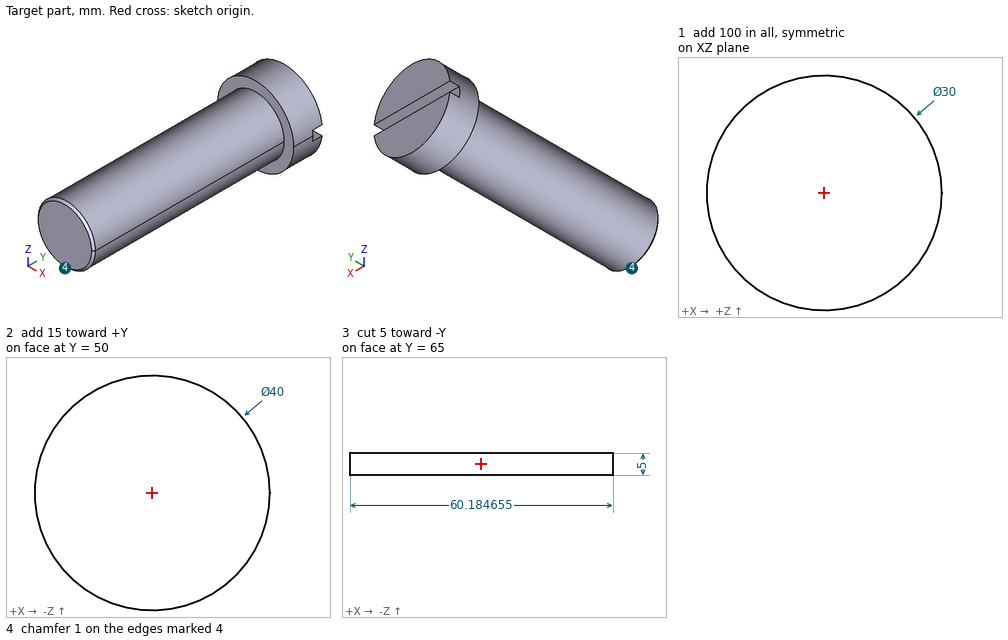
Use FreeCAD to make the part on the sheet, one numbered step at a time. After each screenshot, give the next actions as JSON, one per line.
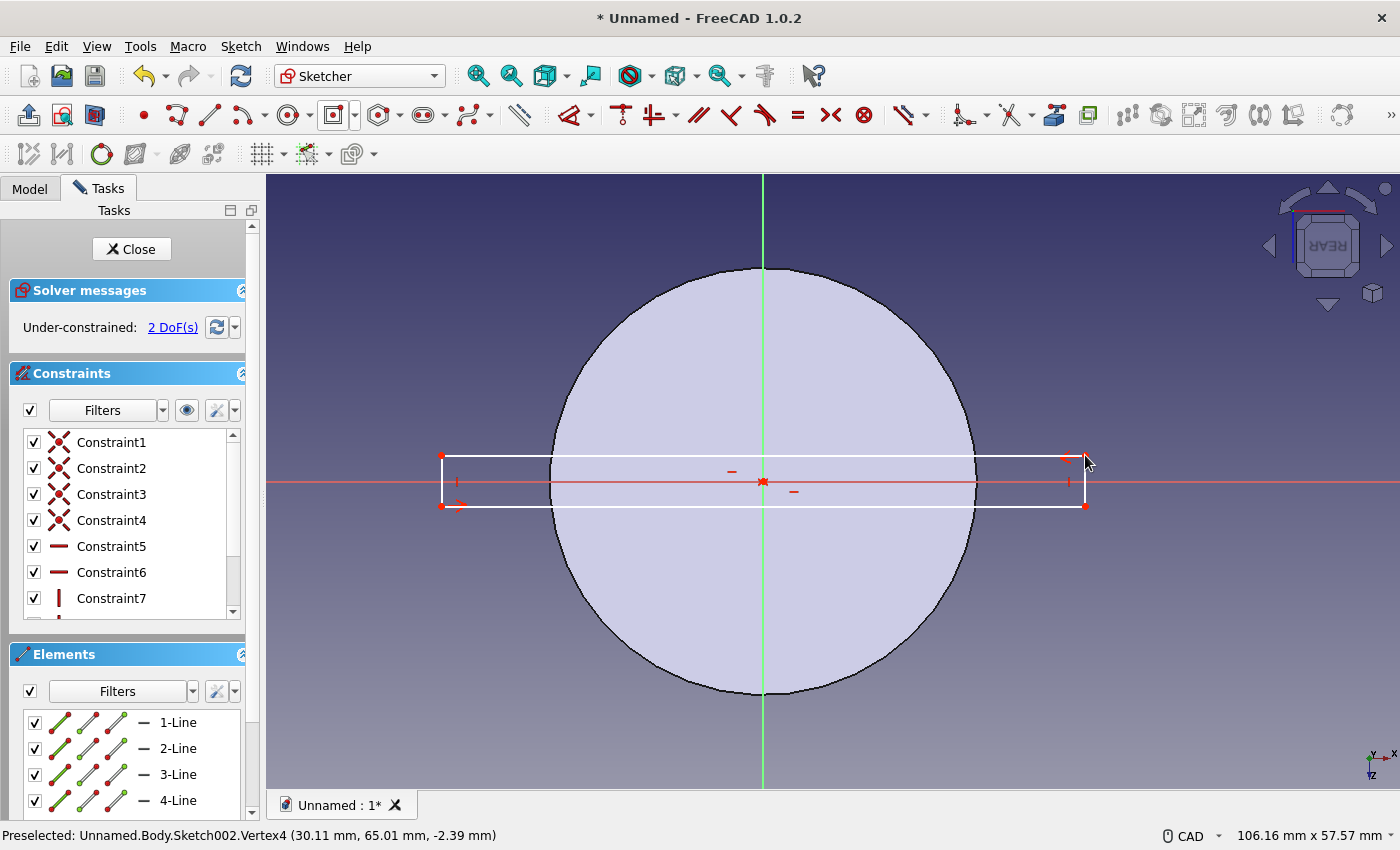
{"action": "left_click", "coordinate": [568, 116]}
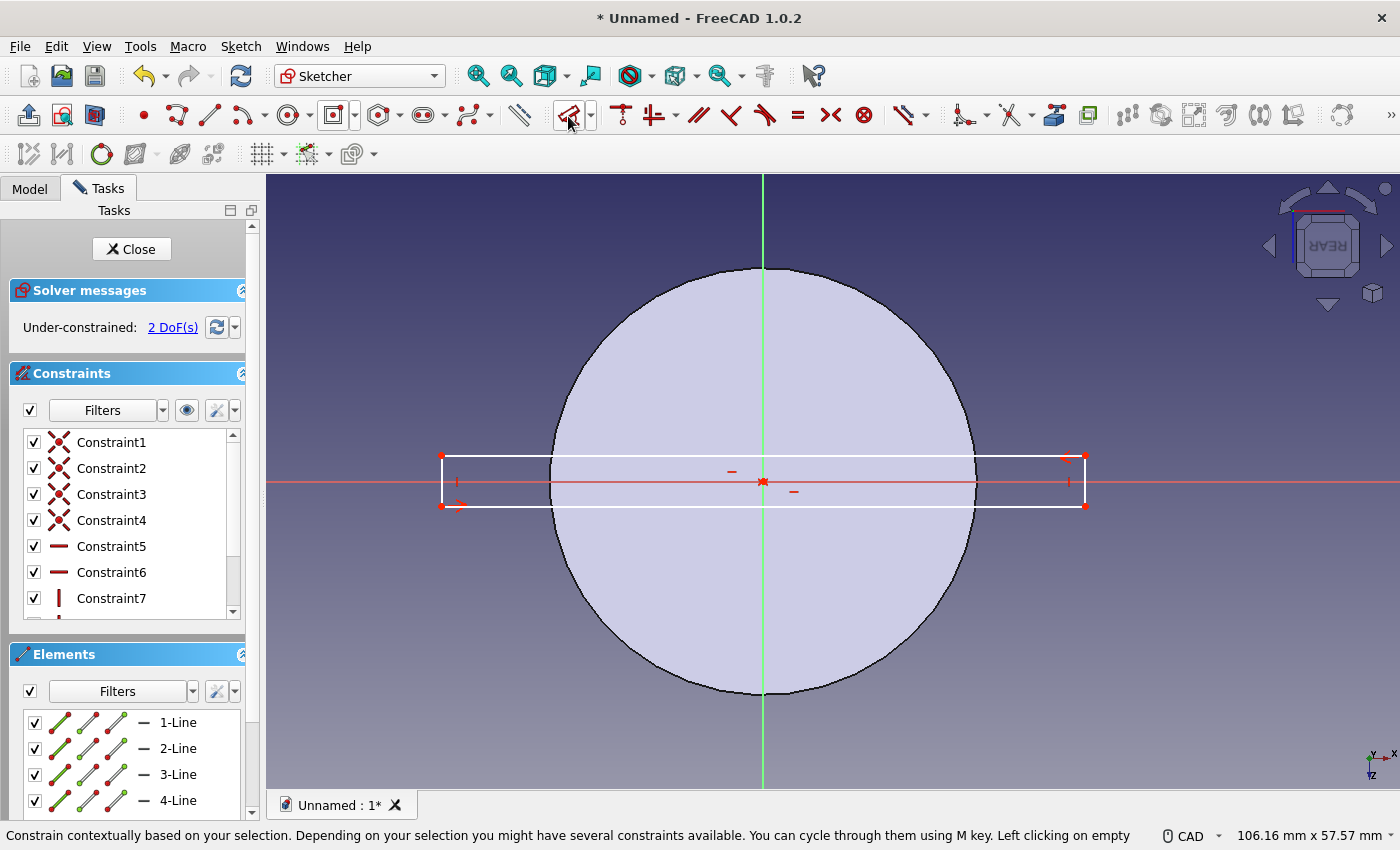
{"action": "scroll", "coordinate": [1085, 492], "scroll_direction": "up", "scroll_amount": 2}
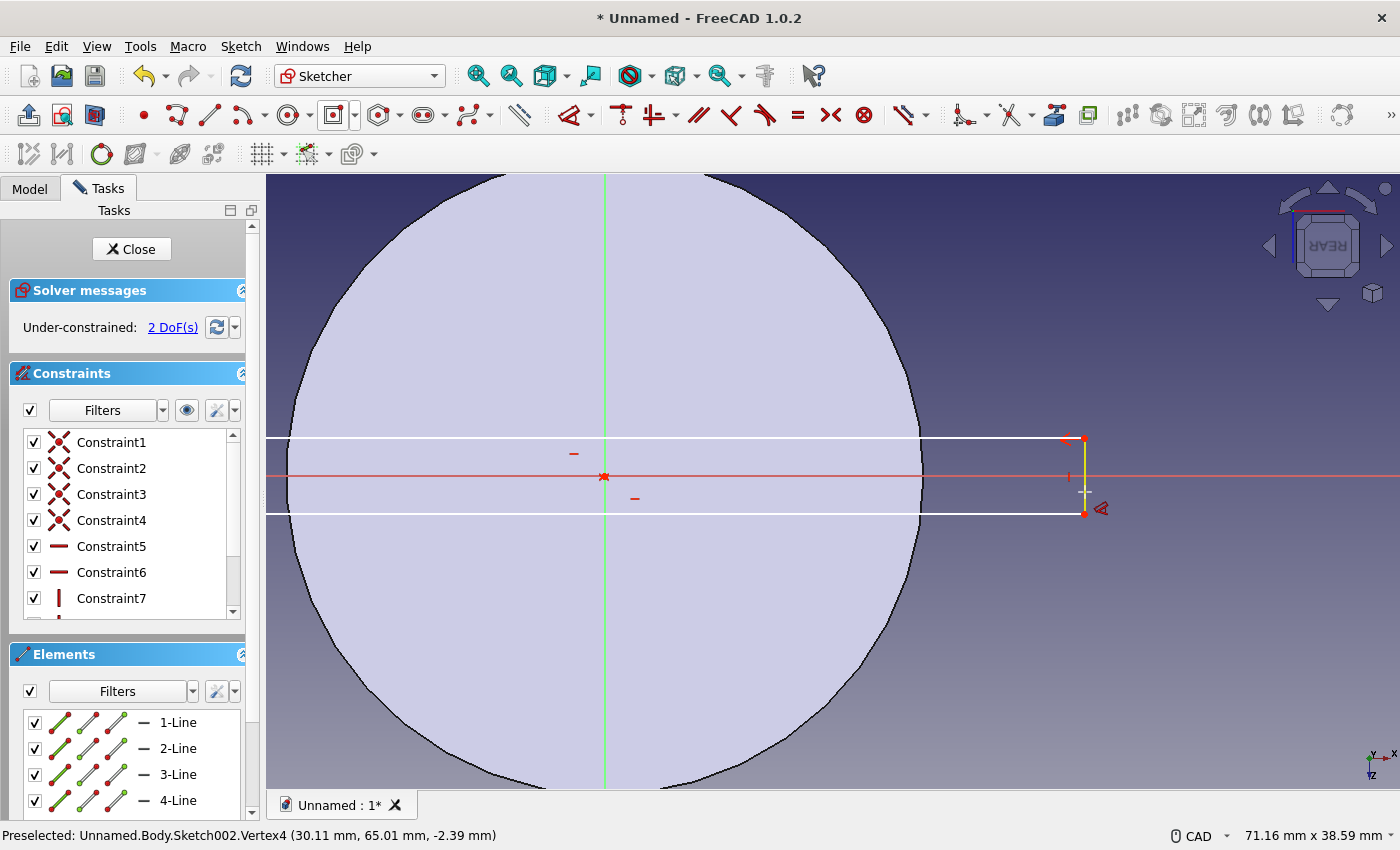
{"action": "left_click", "coordinate": [1085, 491]}
{"action": "left_click", "coordinate": [1119, 459]}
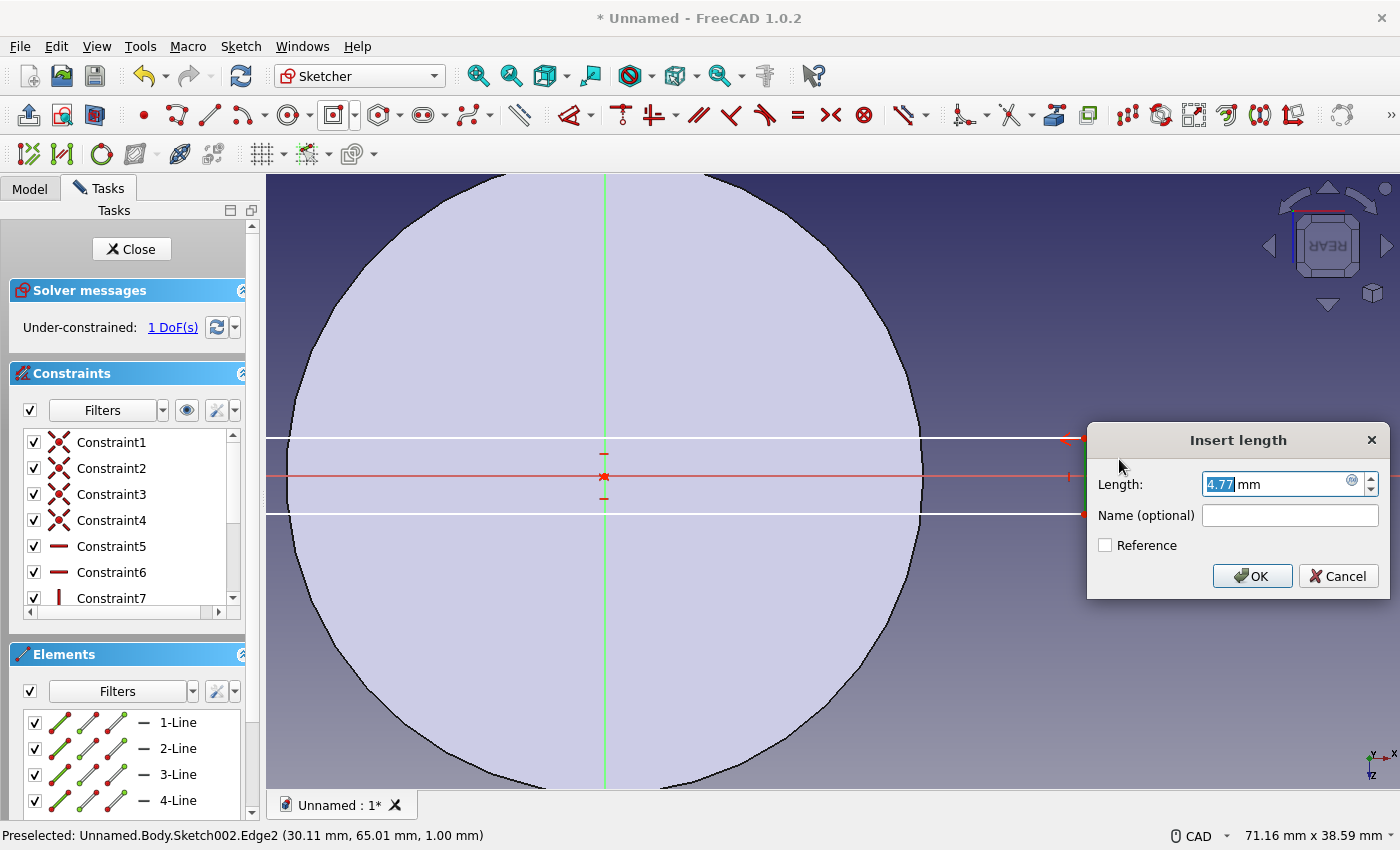
{"action": "type", "text": "5"}
{"action": "key", "text": "Return"}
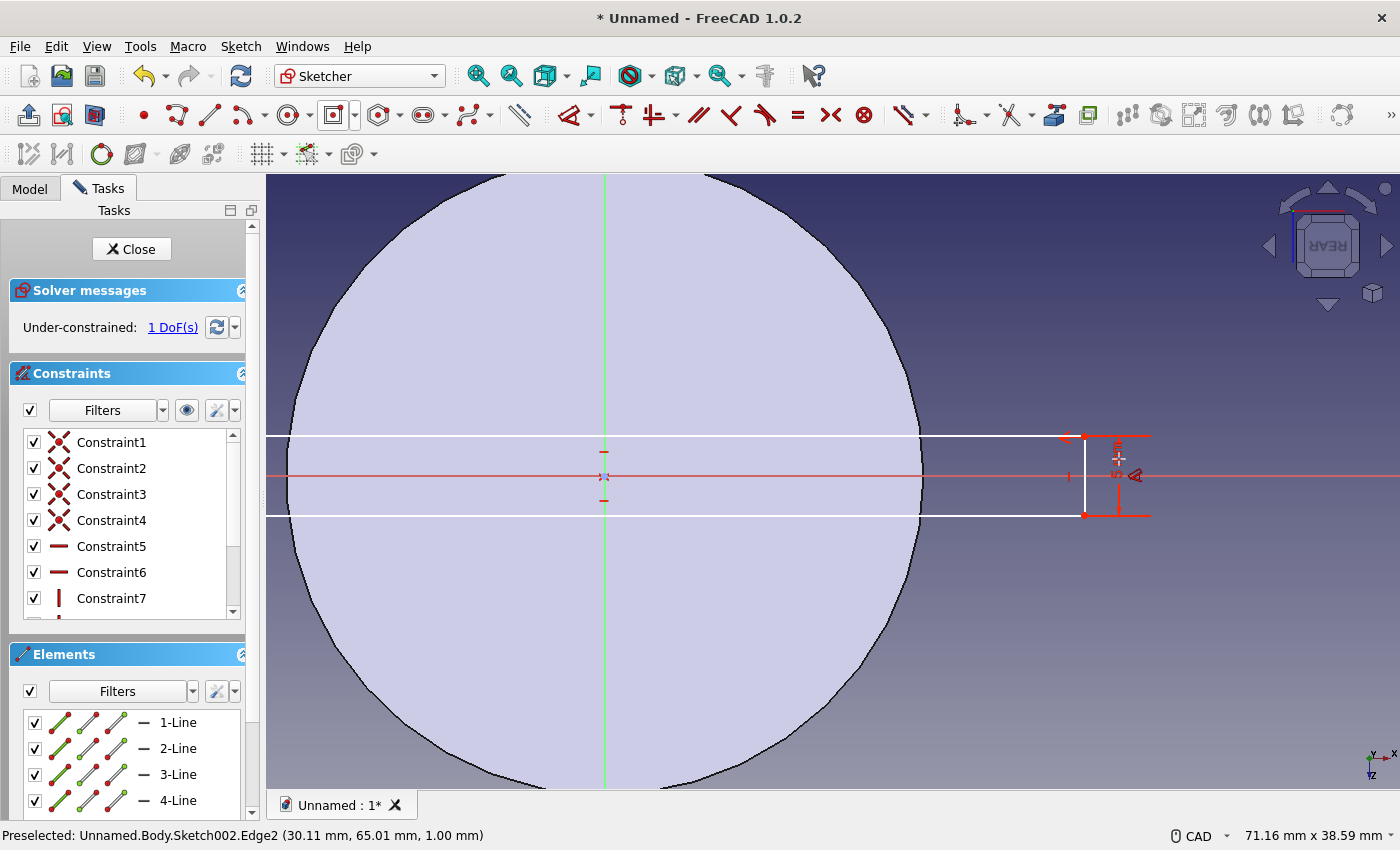
{"action": "left_click", "coordinate": [413, 516]}
{"action": "left_click", "coordinate": [689, 550]}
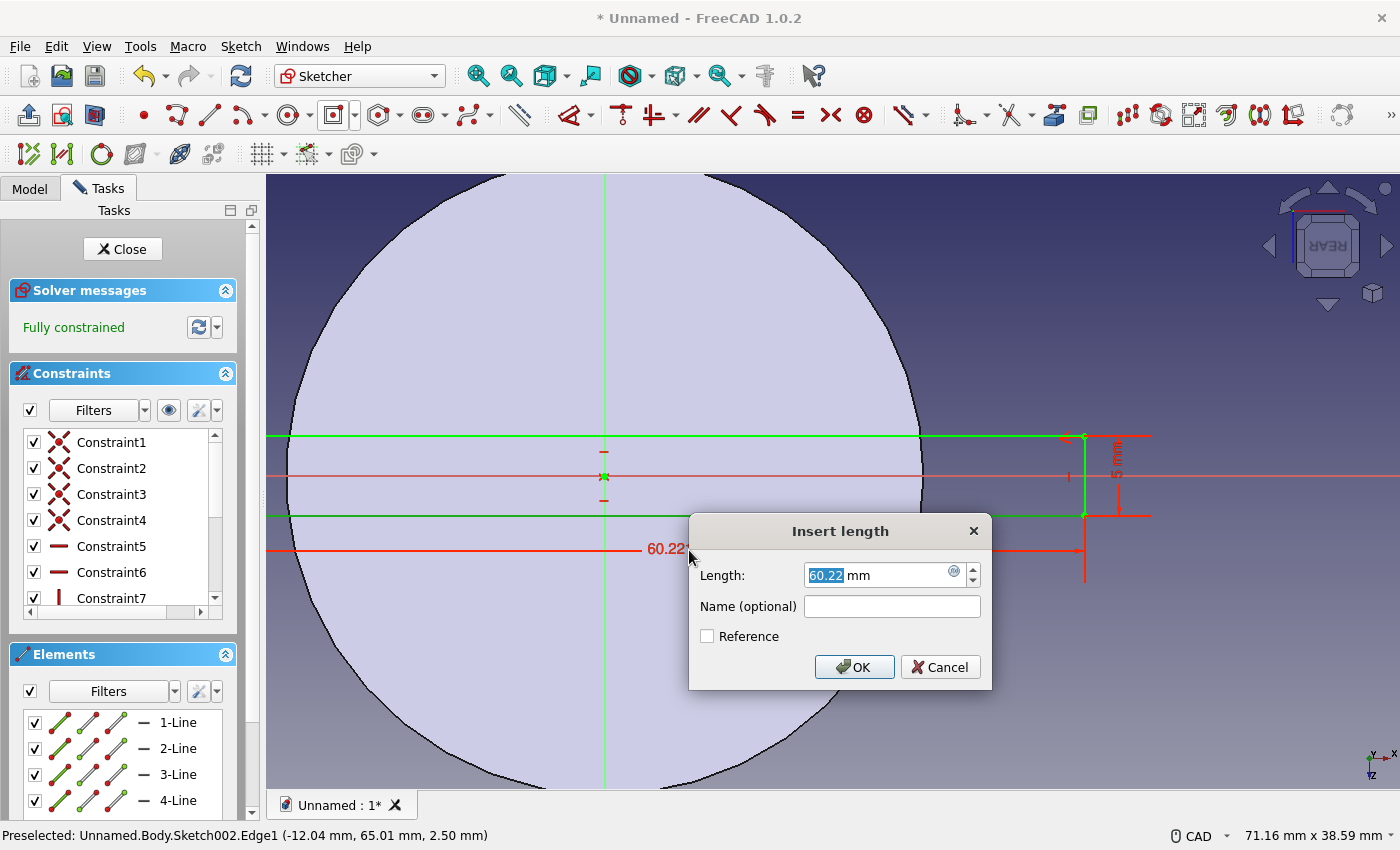
{"action": "type", "text": "60.184655"}
{"action": "key", "text": "Return"}
{"action": "key", "text": "Escape"}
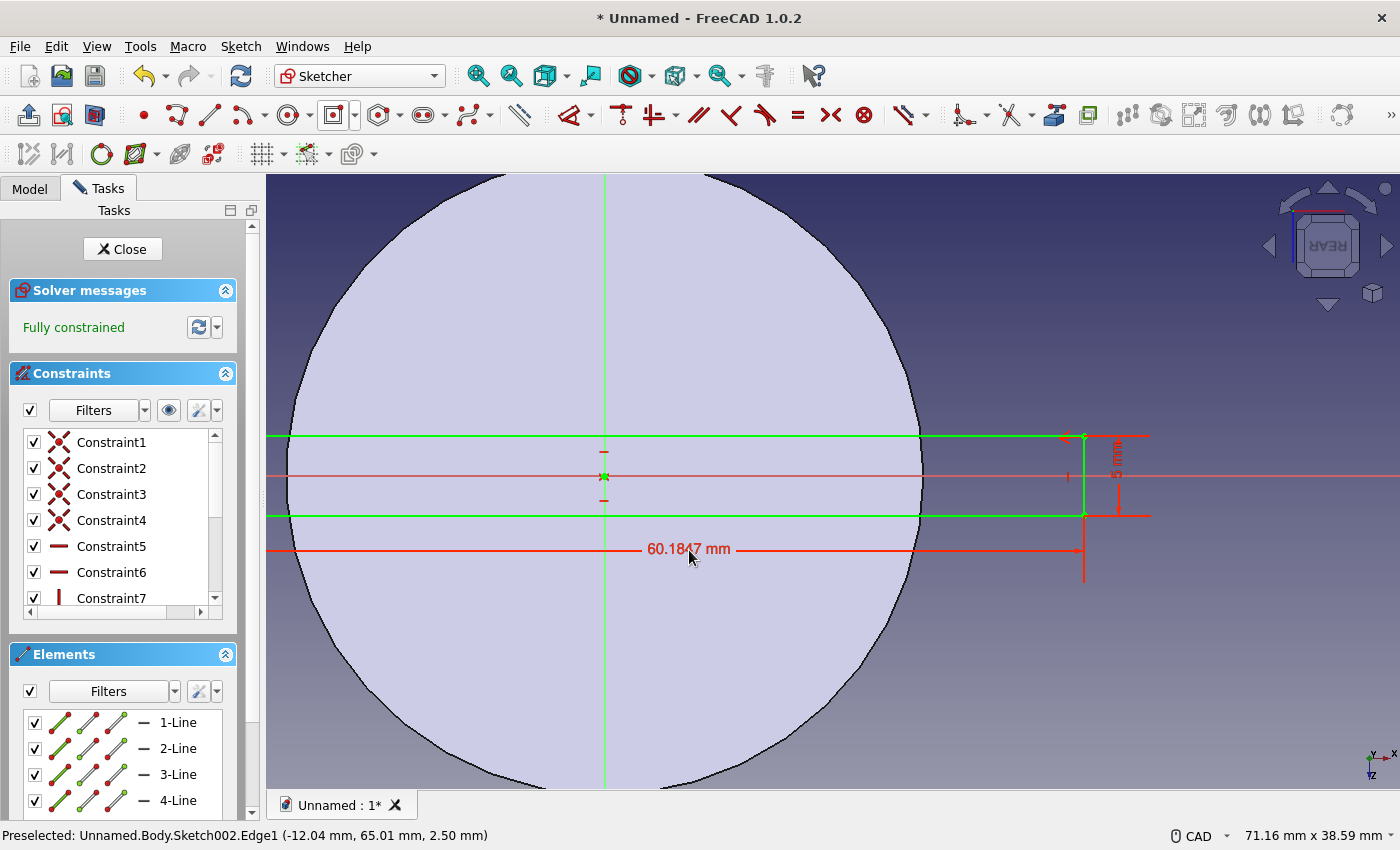
{"action": "left_click", "coordinate": [123, 249]}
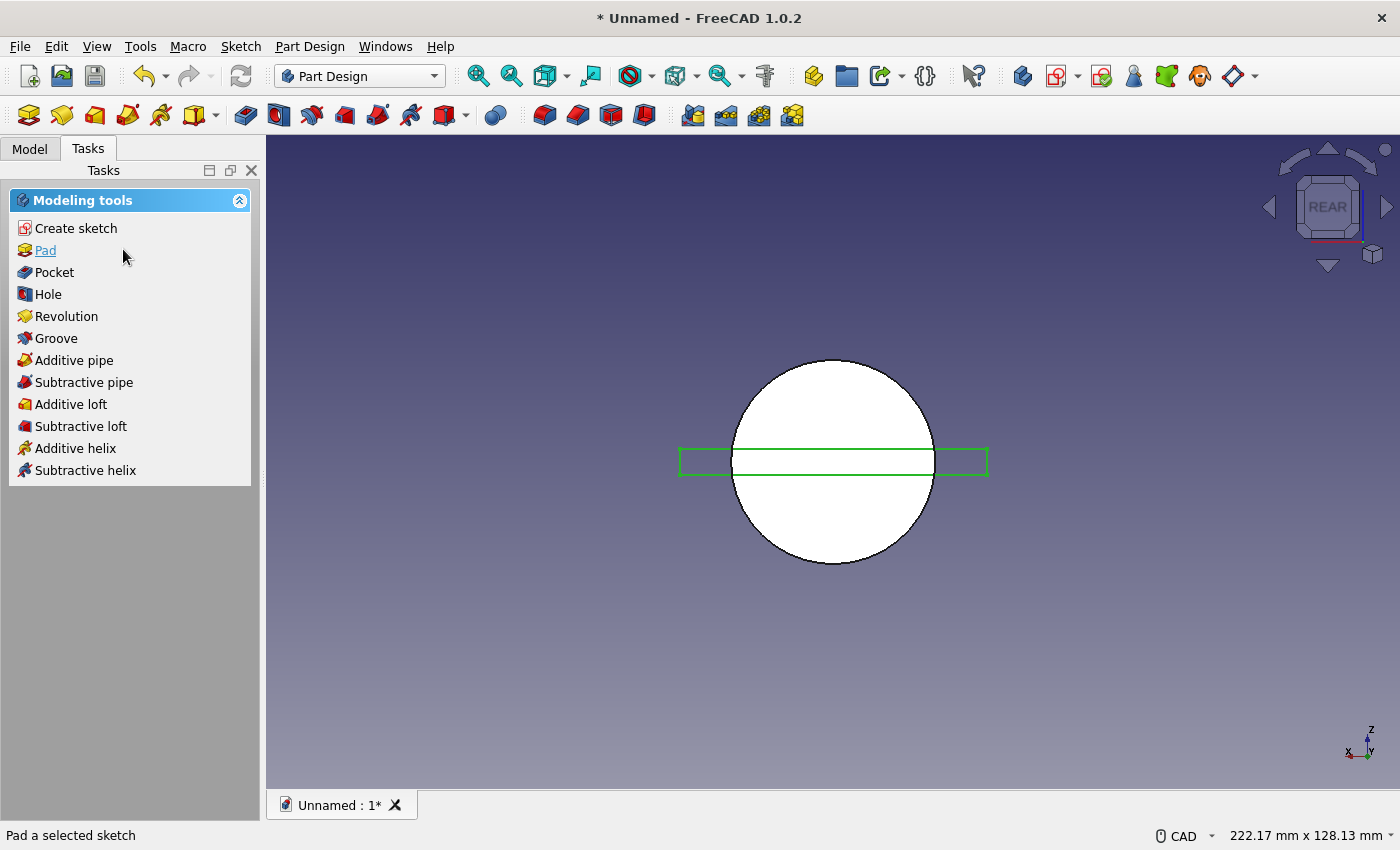
{"action": "left_click", "coordinate": [246, 116]}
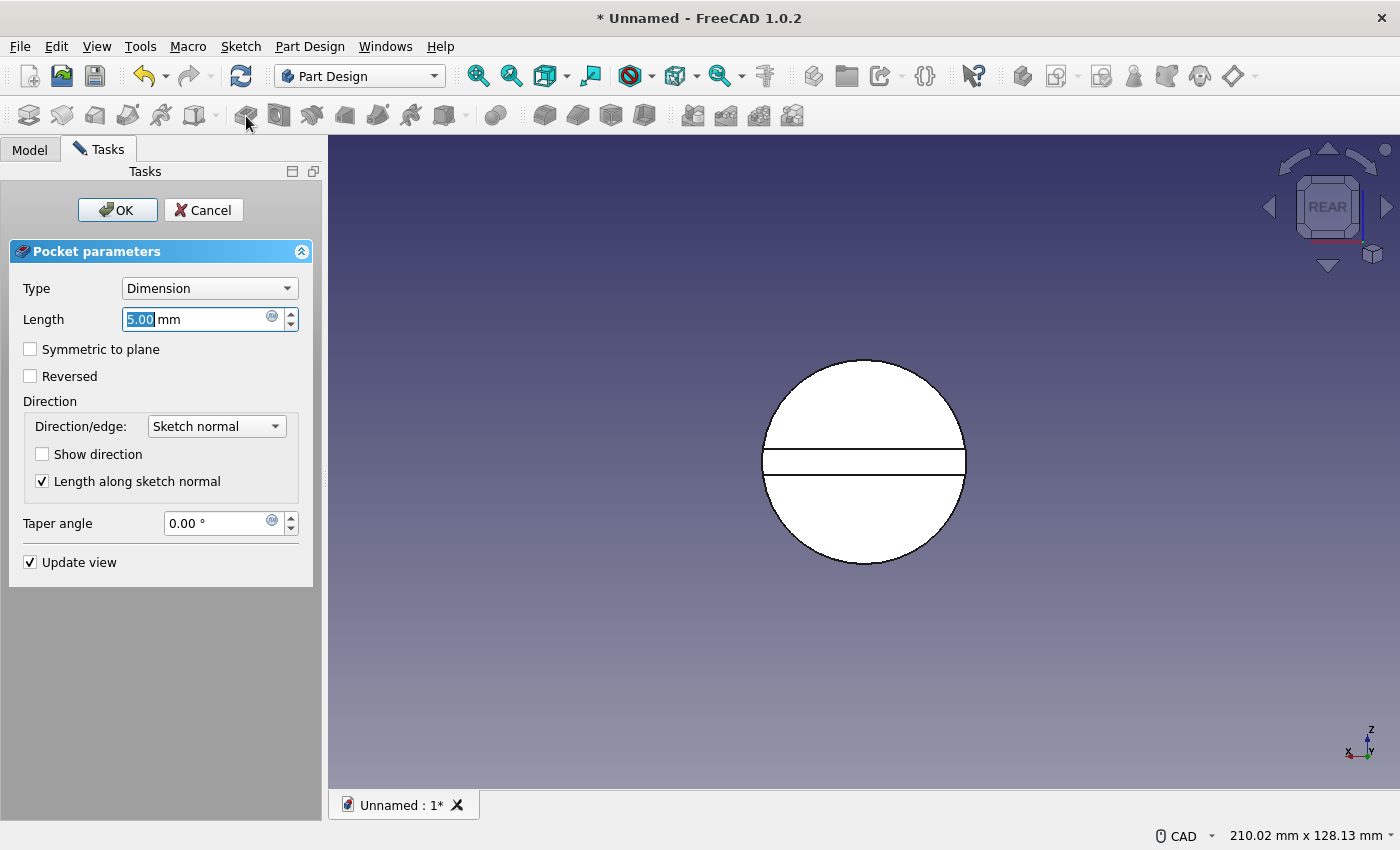
{"action": "type", "text": "5"}
{"action": "key", "text": "Tab"}